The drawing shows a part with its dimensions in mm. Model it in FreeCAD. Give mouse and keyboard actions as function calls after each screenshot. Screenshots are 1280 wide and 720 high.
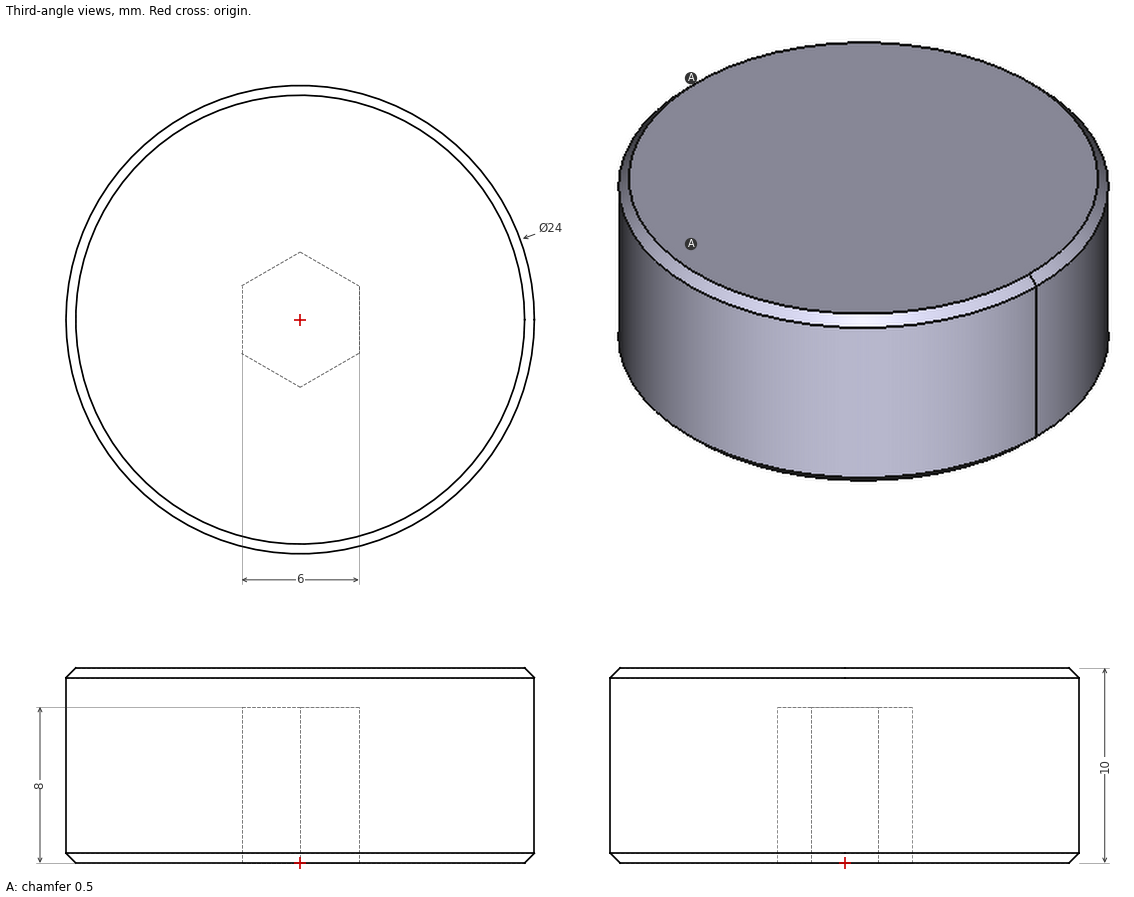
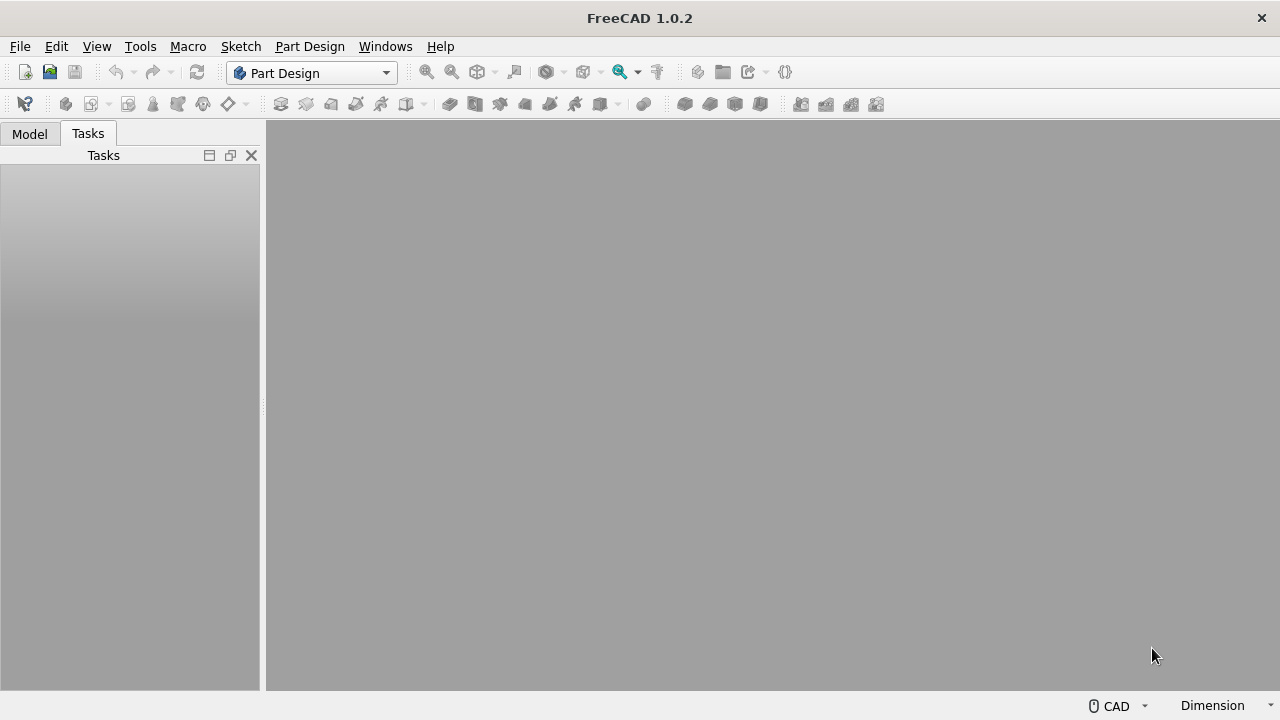
click(25, 72)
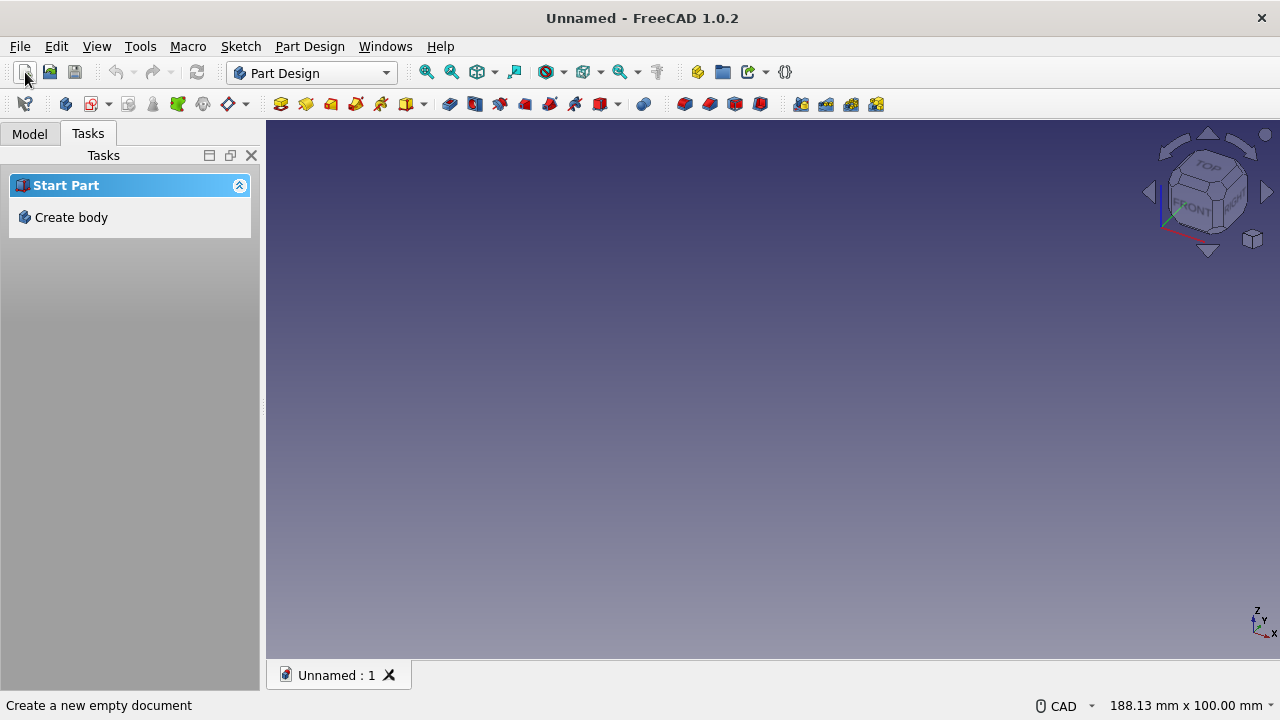
click(90, 104)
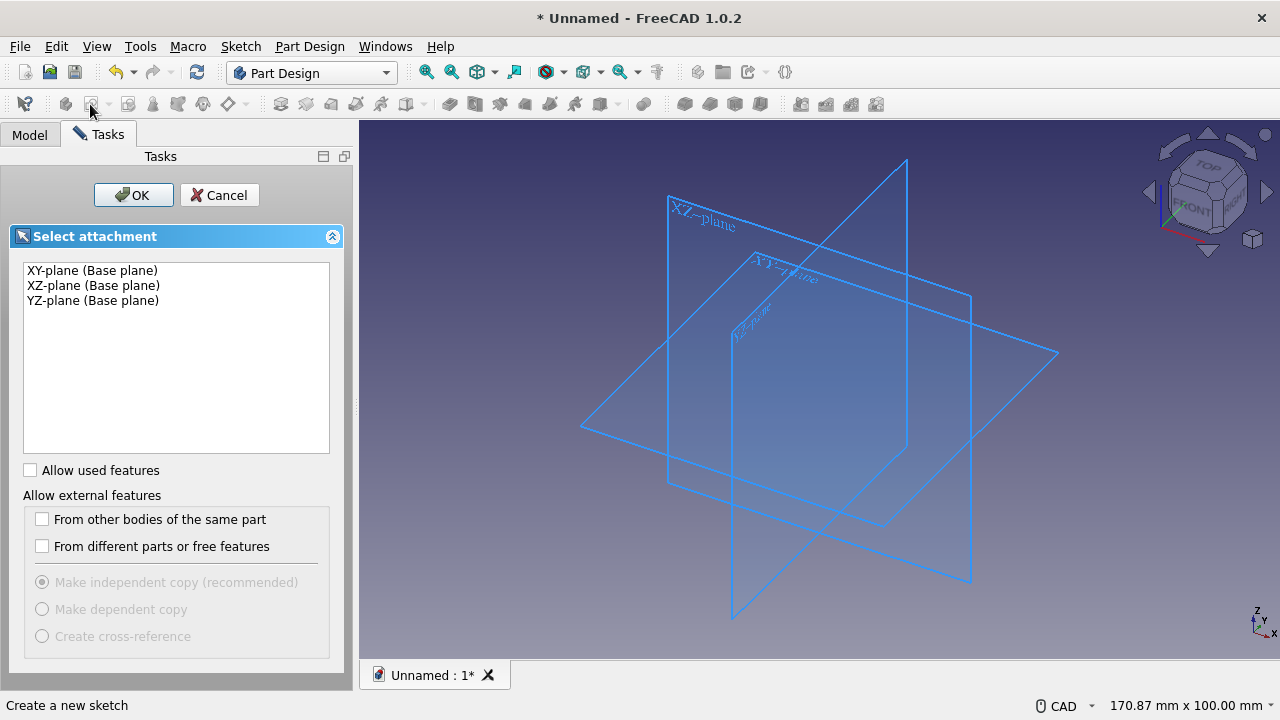
click(84, 270)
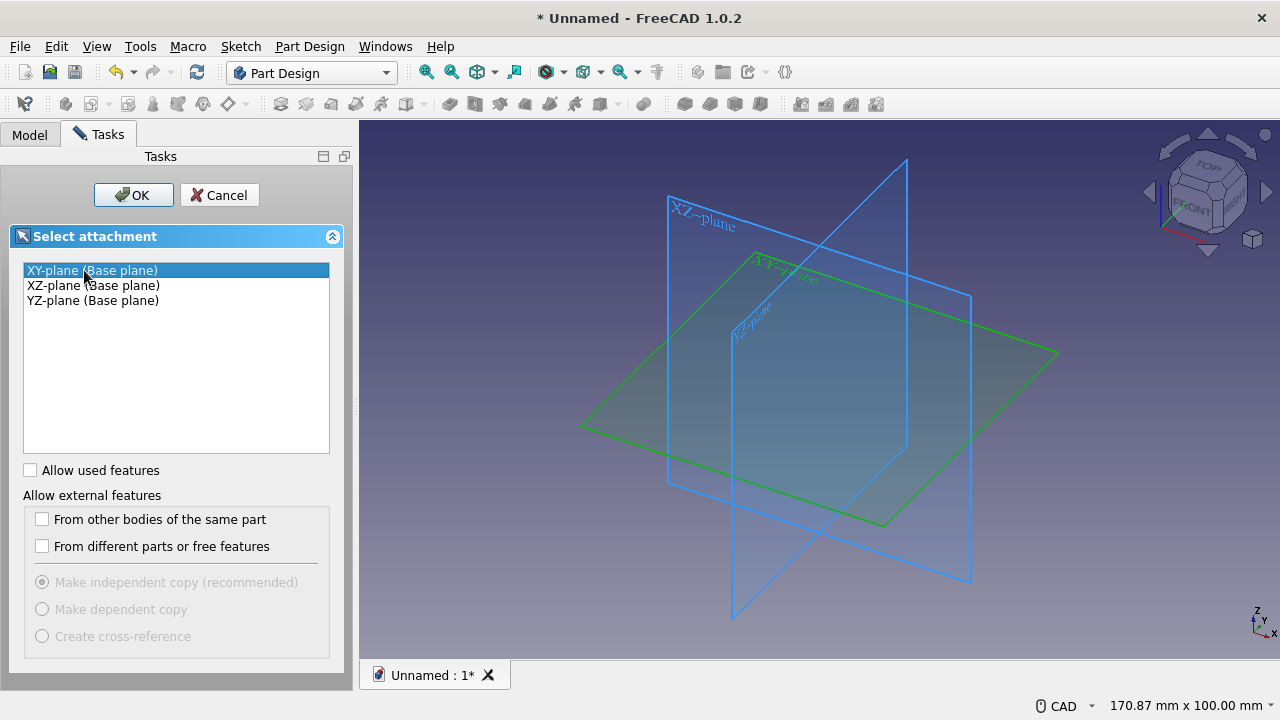
click(134, 195)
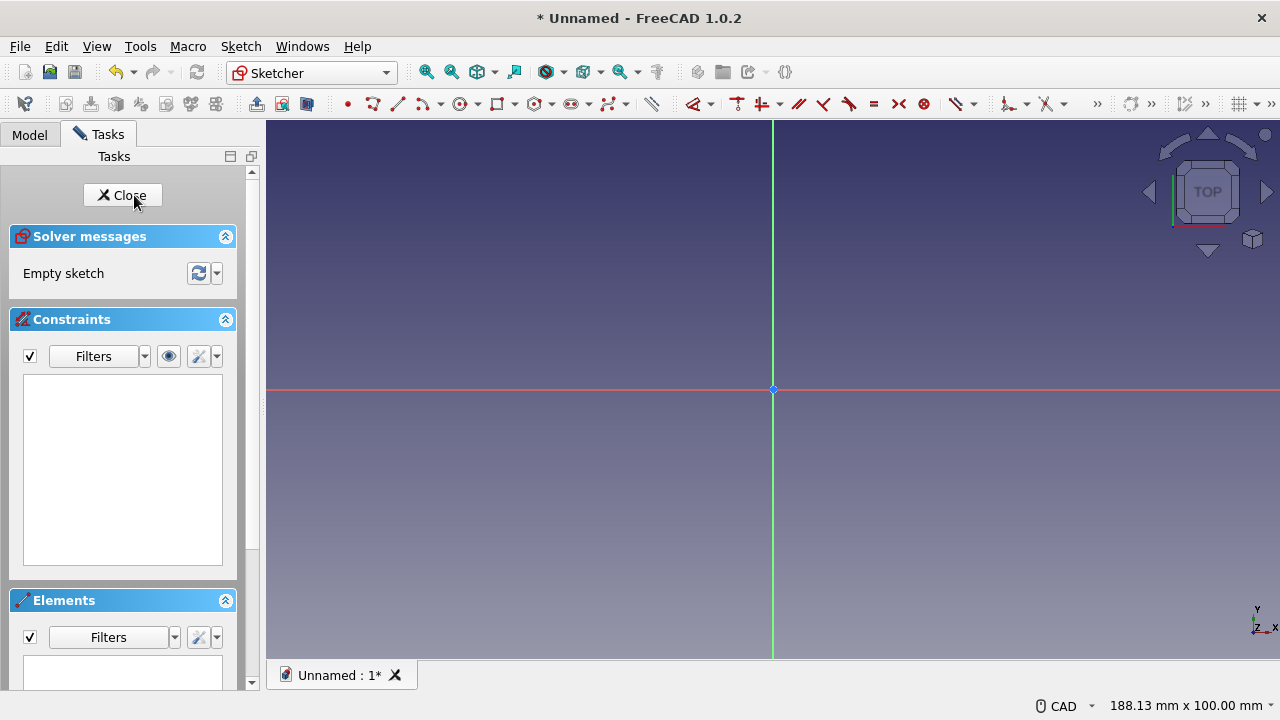
scroll(813, 390, up, 5)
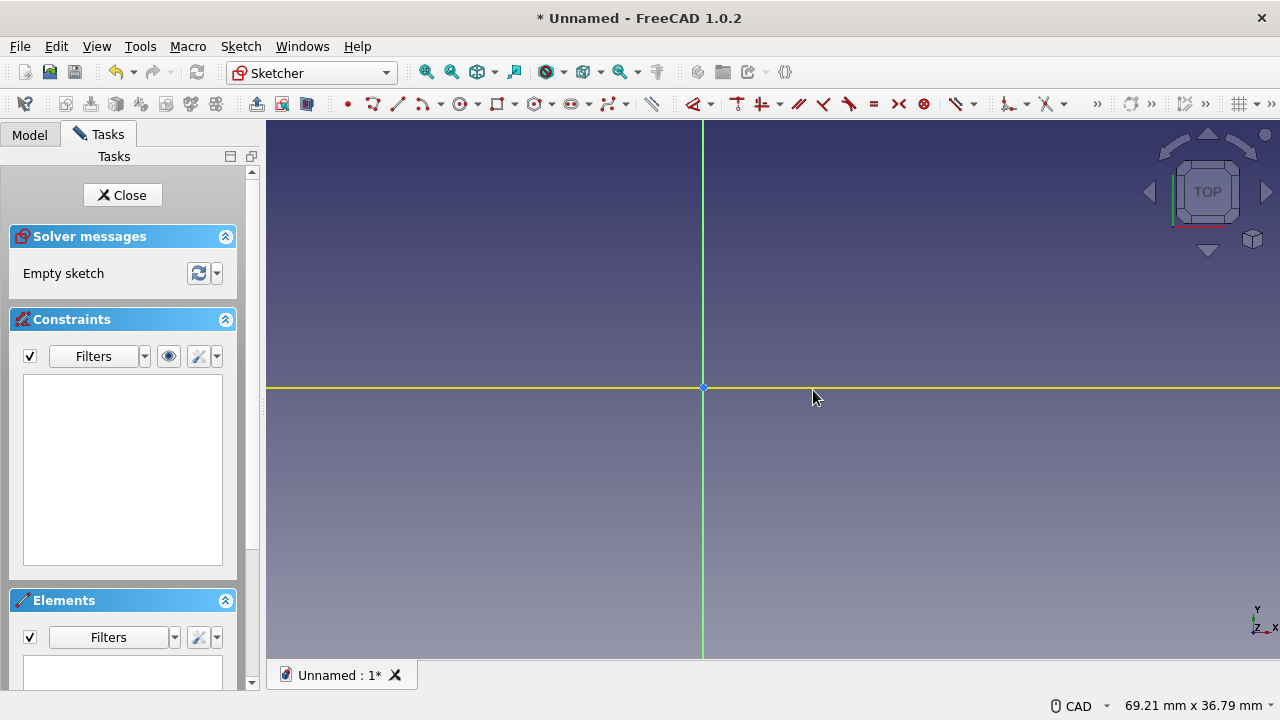
click(460, 104)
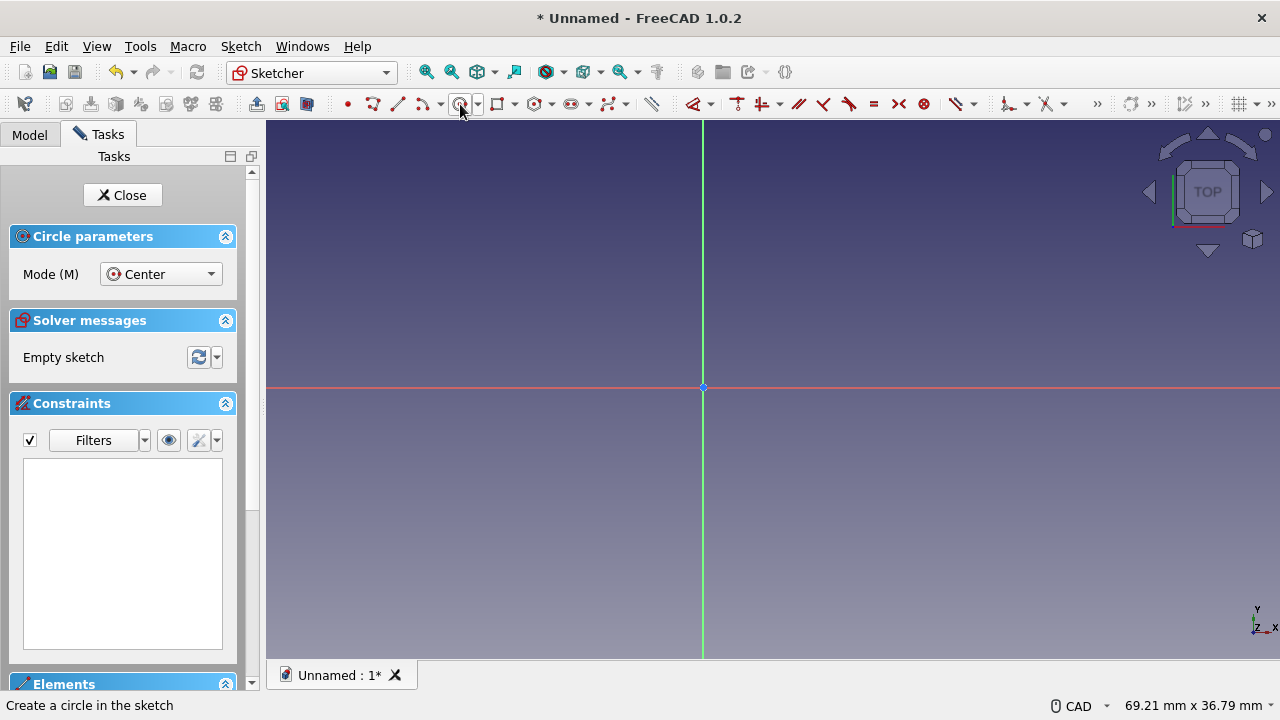
click(703, 388)
click(828, 263)
key(Escape)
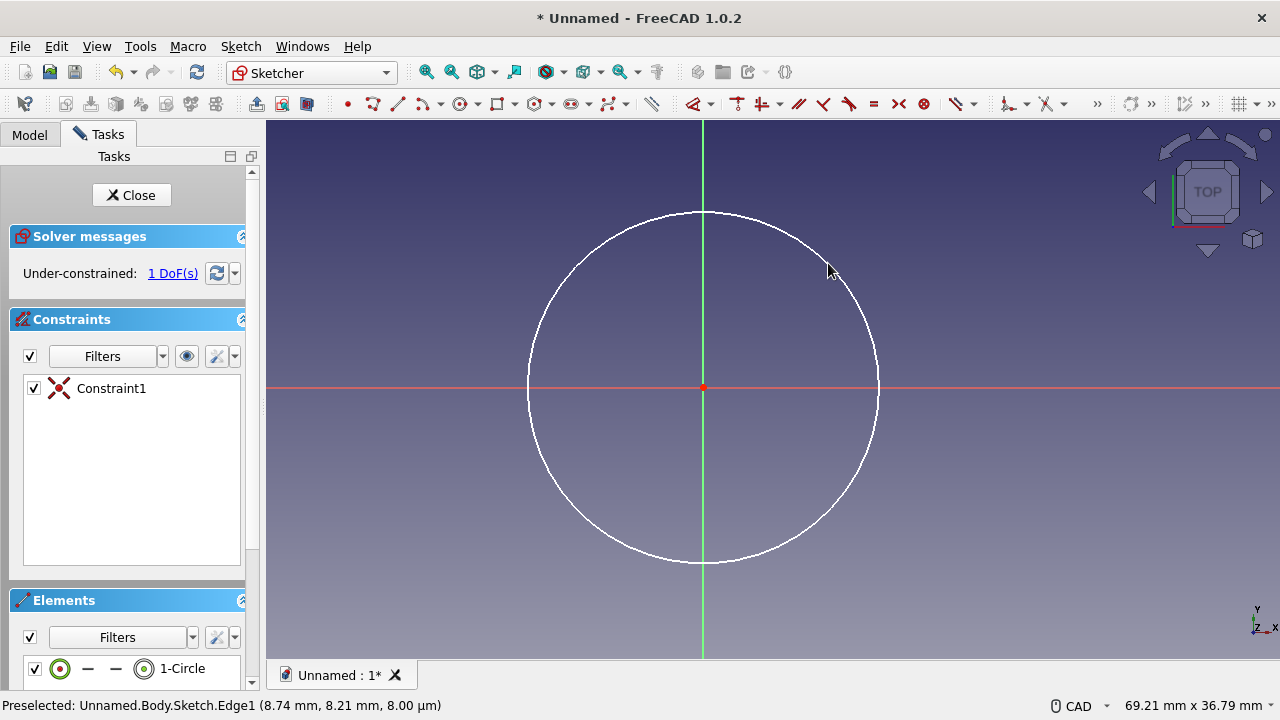
click(827, 263)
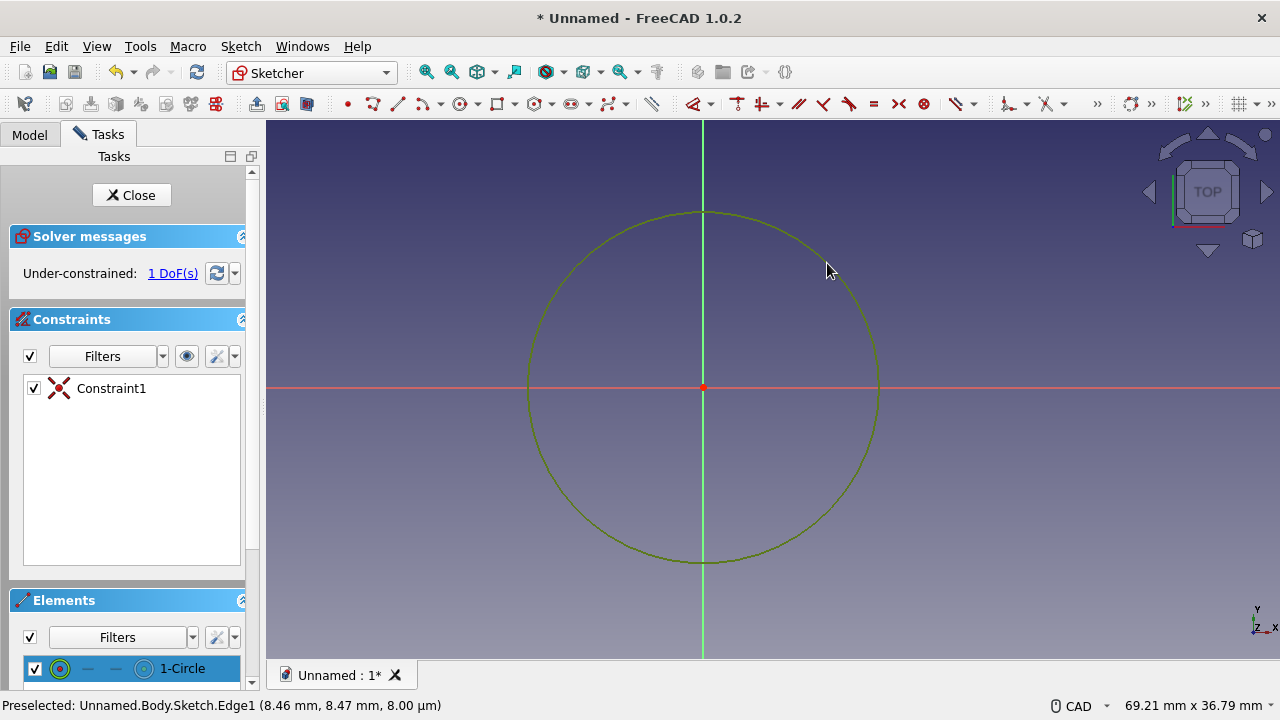
click(710, 104)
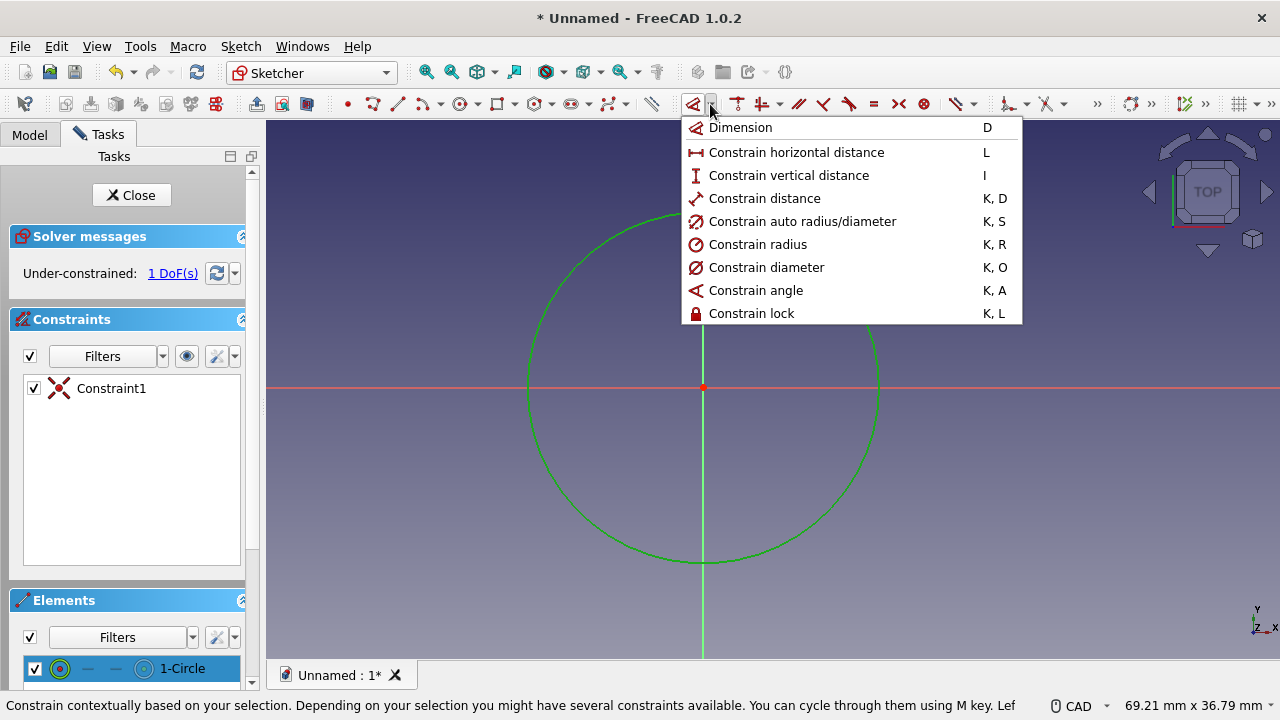
click(852, 268)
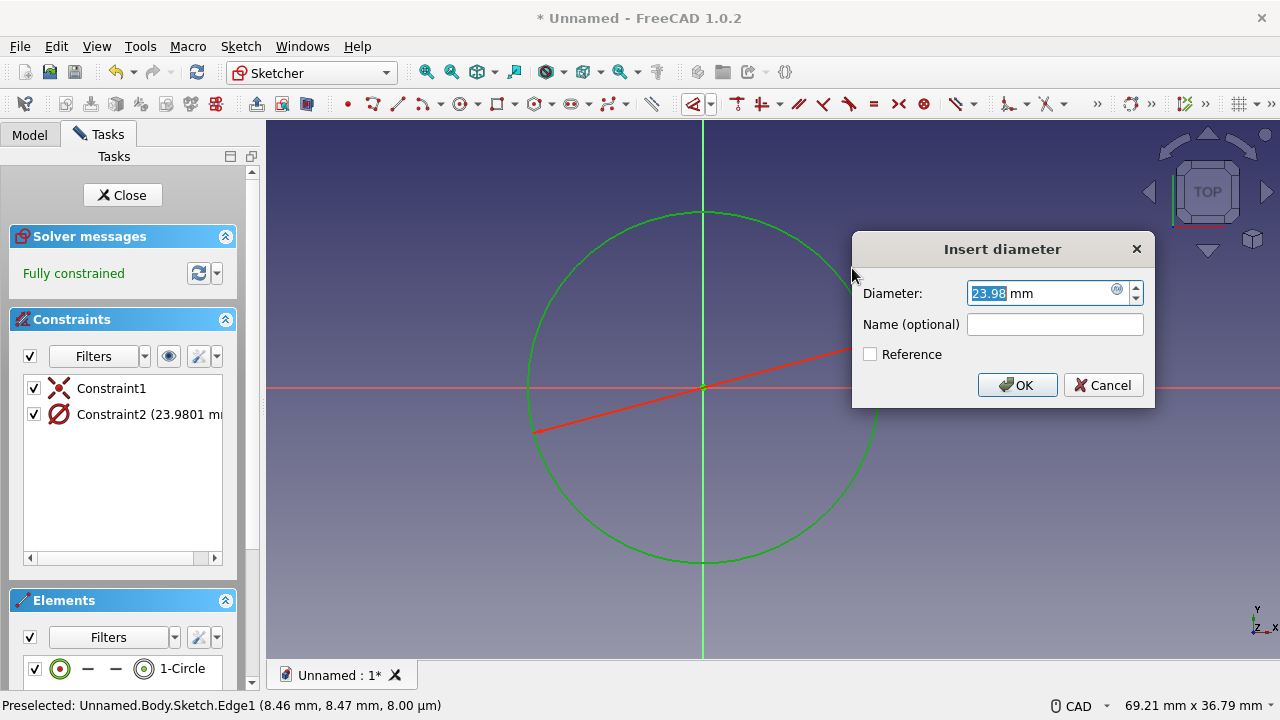
text(24)
key(Return)